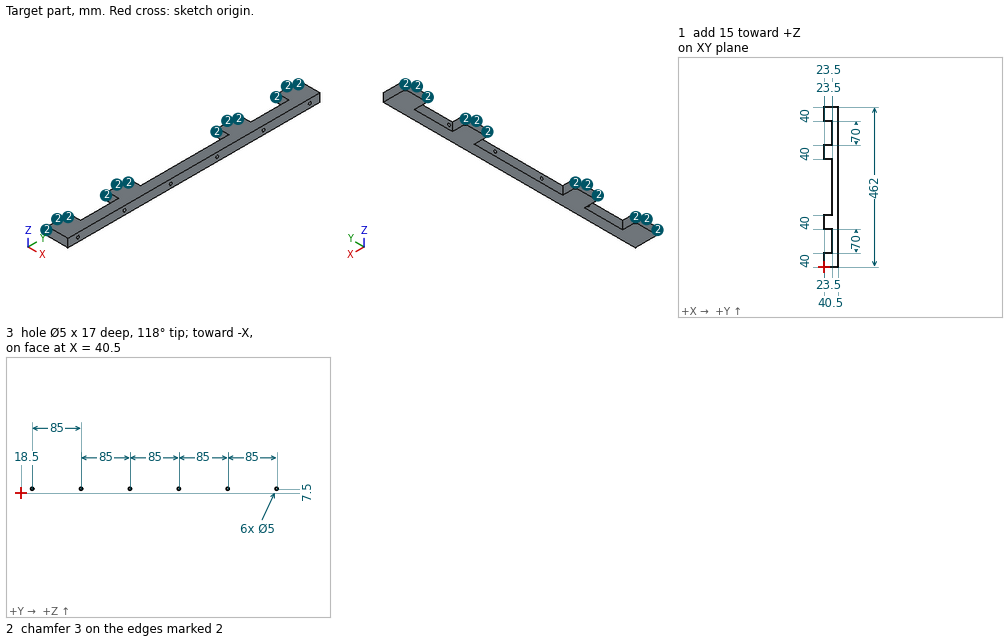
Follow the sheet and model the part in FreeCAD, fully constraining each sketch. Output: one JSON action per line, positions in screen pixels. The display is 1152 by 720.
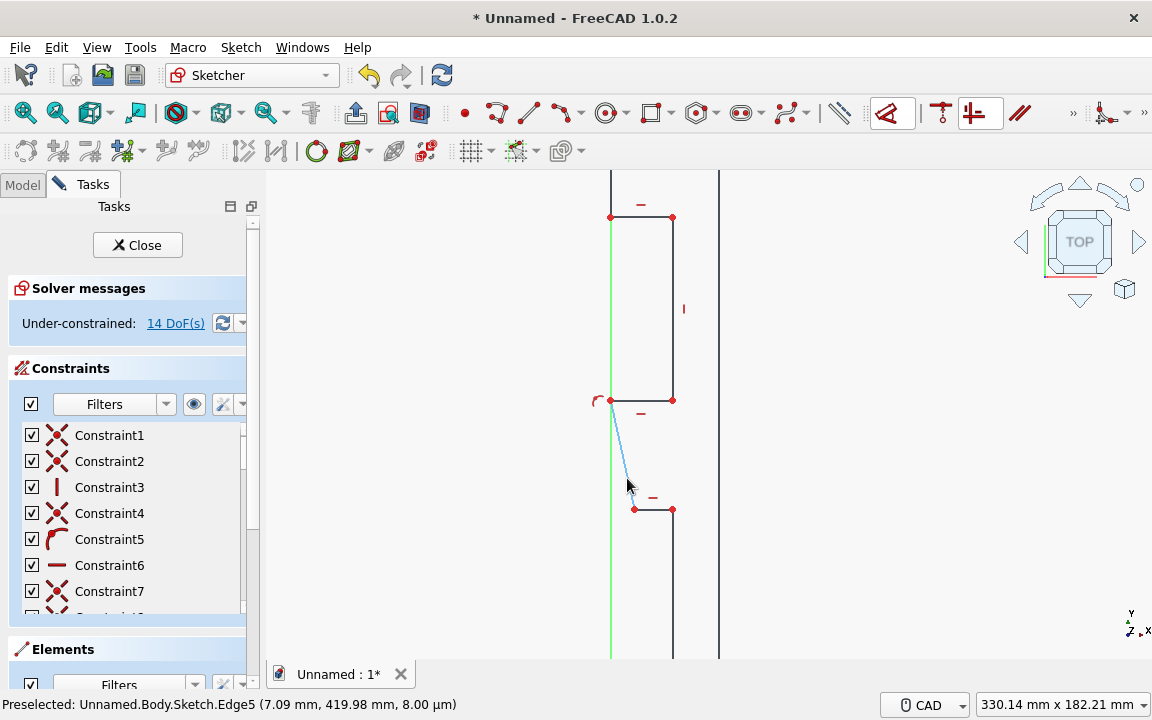
{"action": "left_click", "coordinate": [627, 477]}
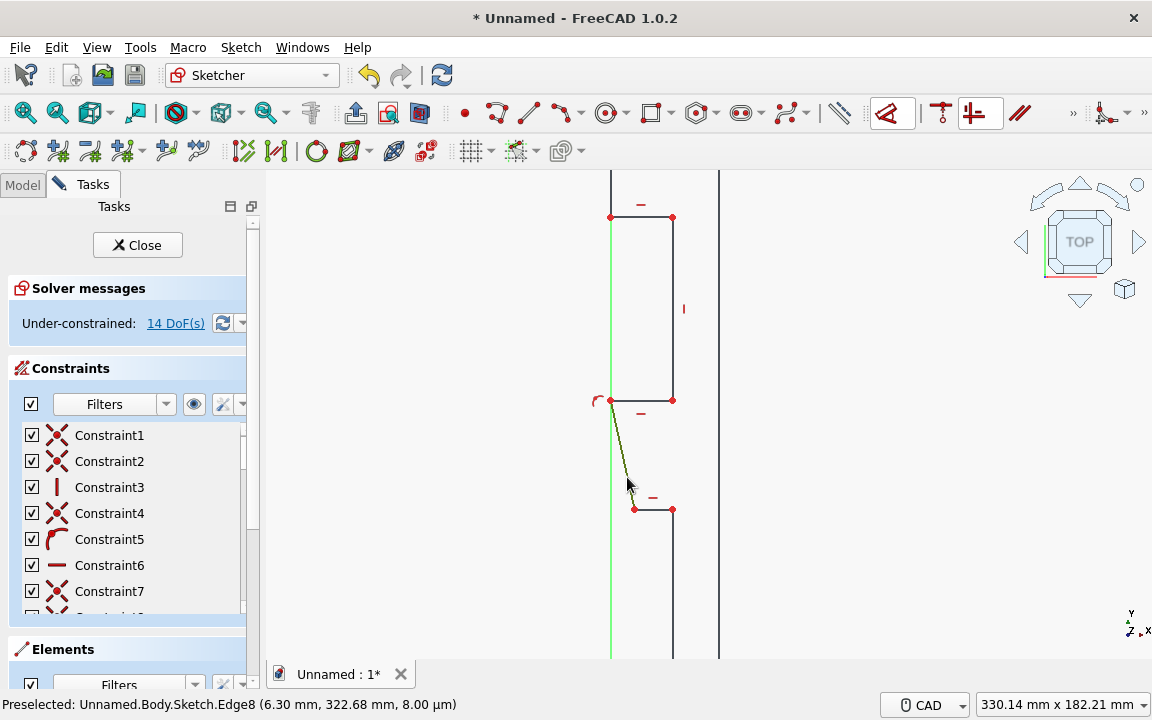
{"action": "key", "text": "v"}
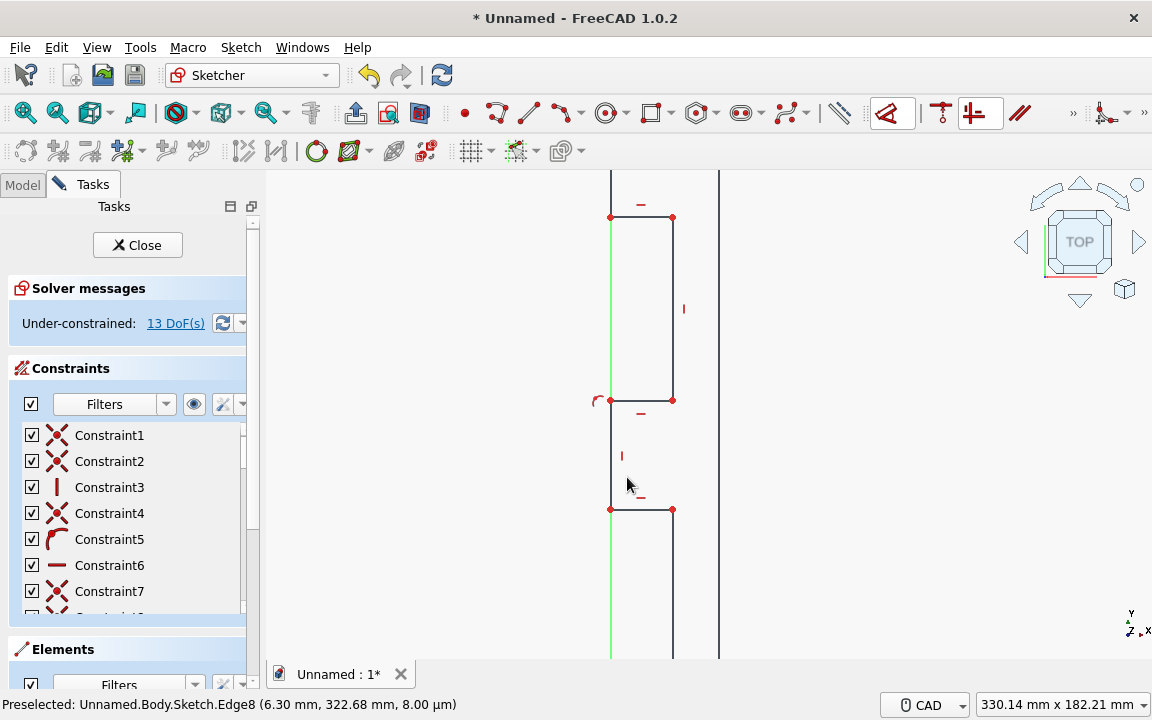
{"action": "scroll", "coordinate": [632, 313], "scroll_direction": "down", "scroll_amount": 7}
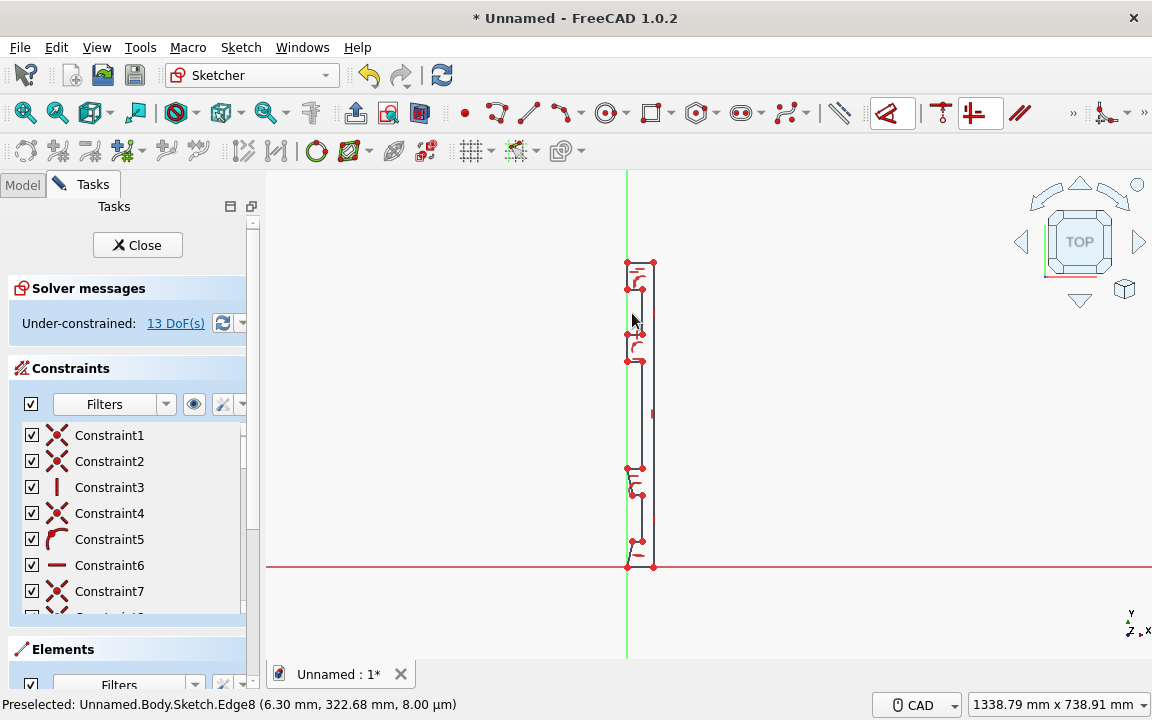
{"action": "scroll", "coordinate": [631, 487], "scroll_direction": "up", "scroll_amount": 7}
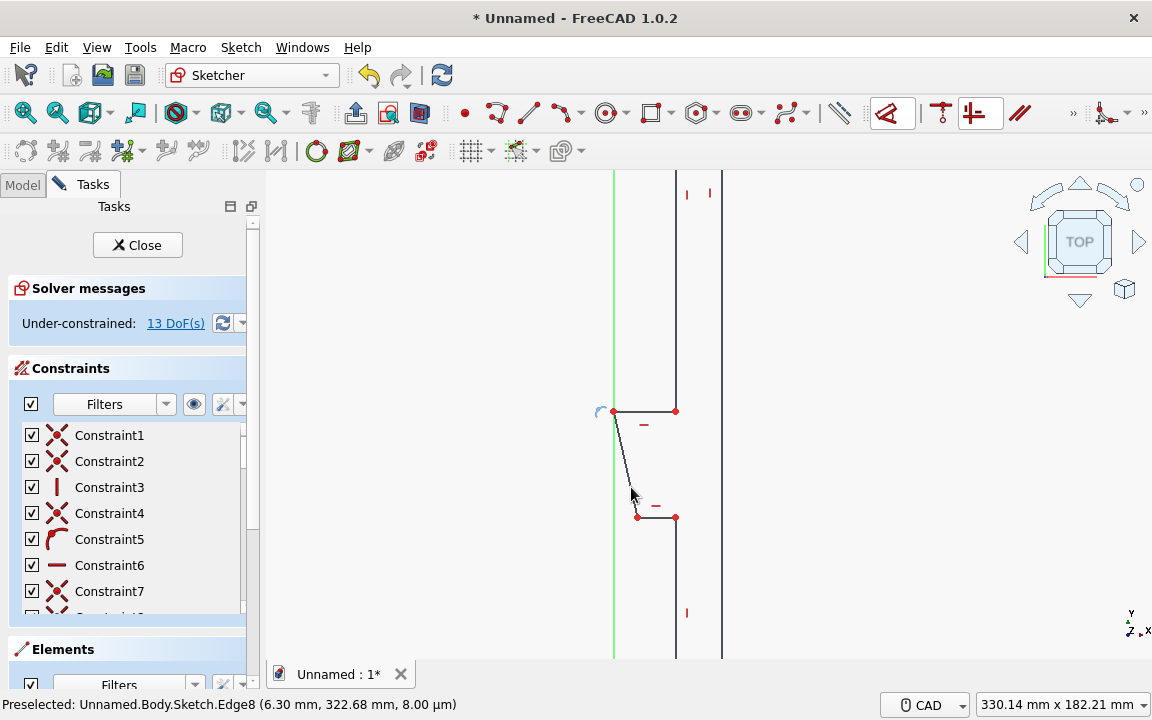
{"action": "left_click", "coordinate": [631, 486]}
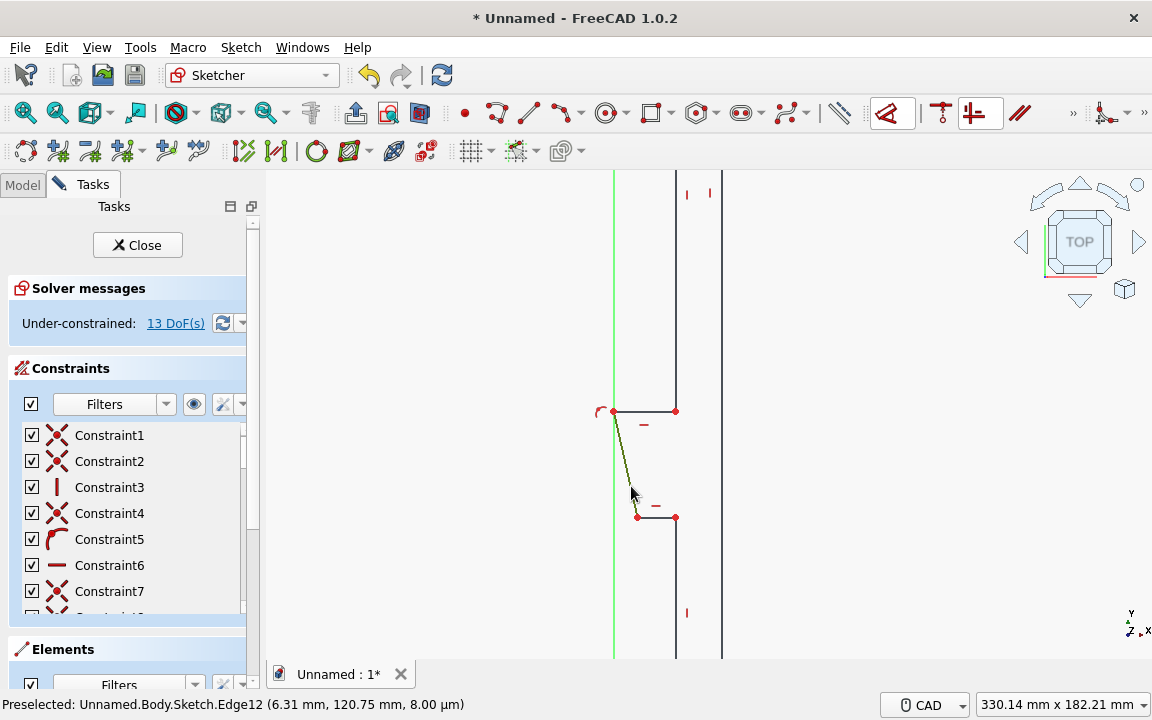
{"action": "left_click", "coordinate": [998, 114]}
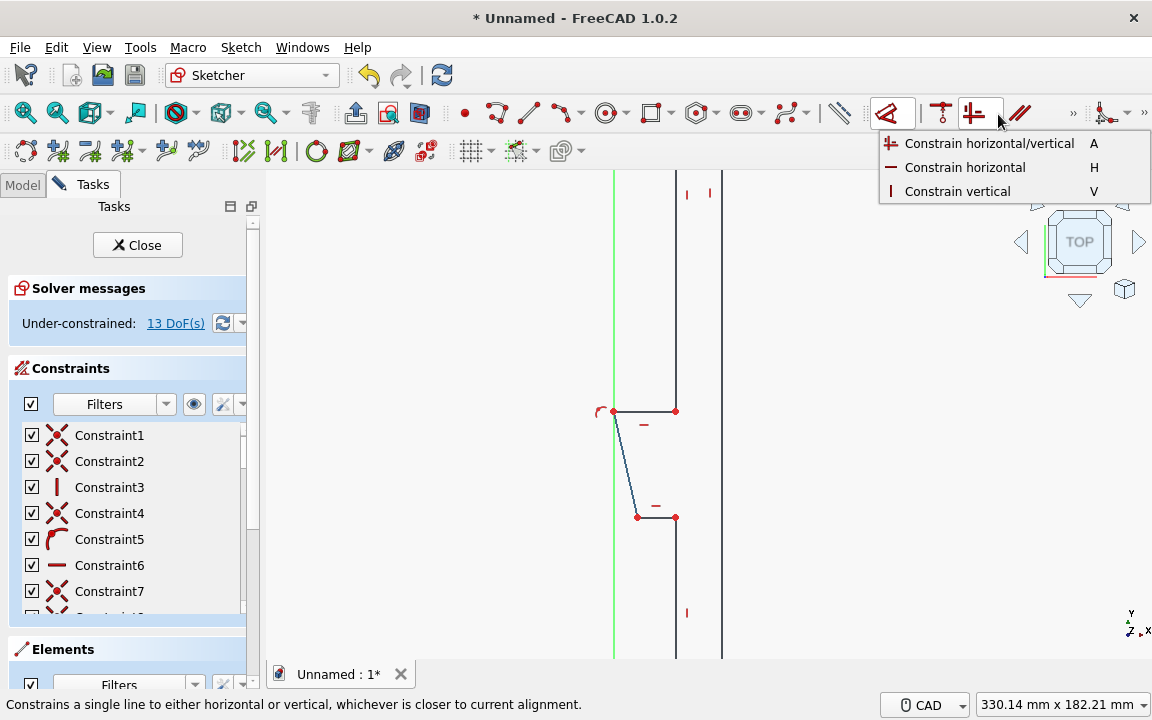
{"action": "left_click", "coordinate": [1015, 191]}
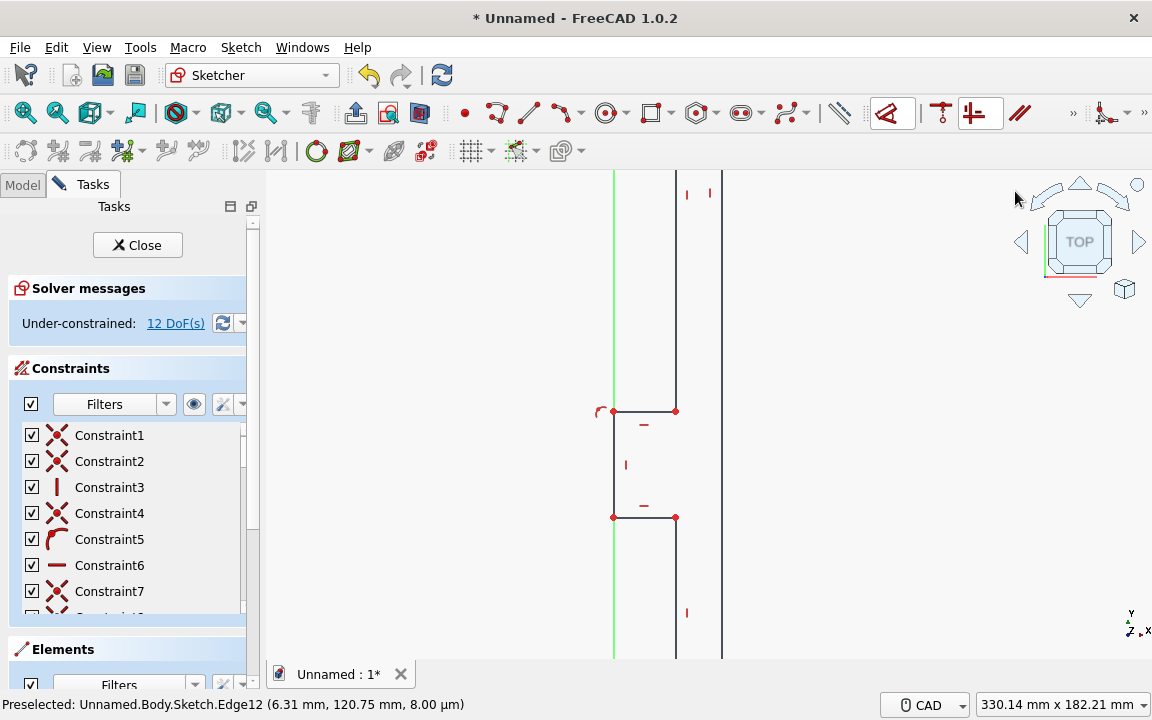
{"action": "scroll", "coordinate": [631, 488], "scroll_direction": "down", "scroll_amount": 7}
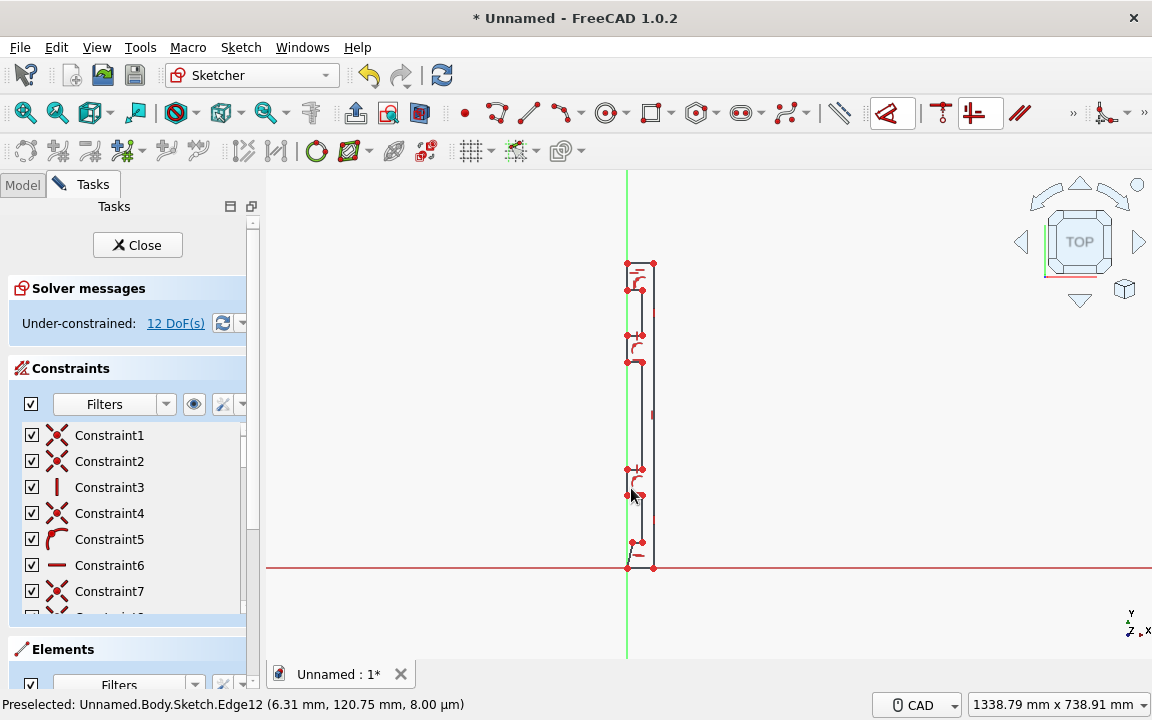
{"action": "scroll", "coordinate": [631, 550], "scroll_direction": "up", "scroll_amount": 7}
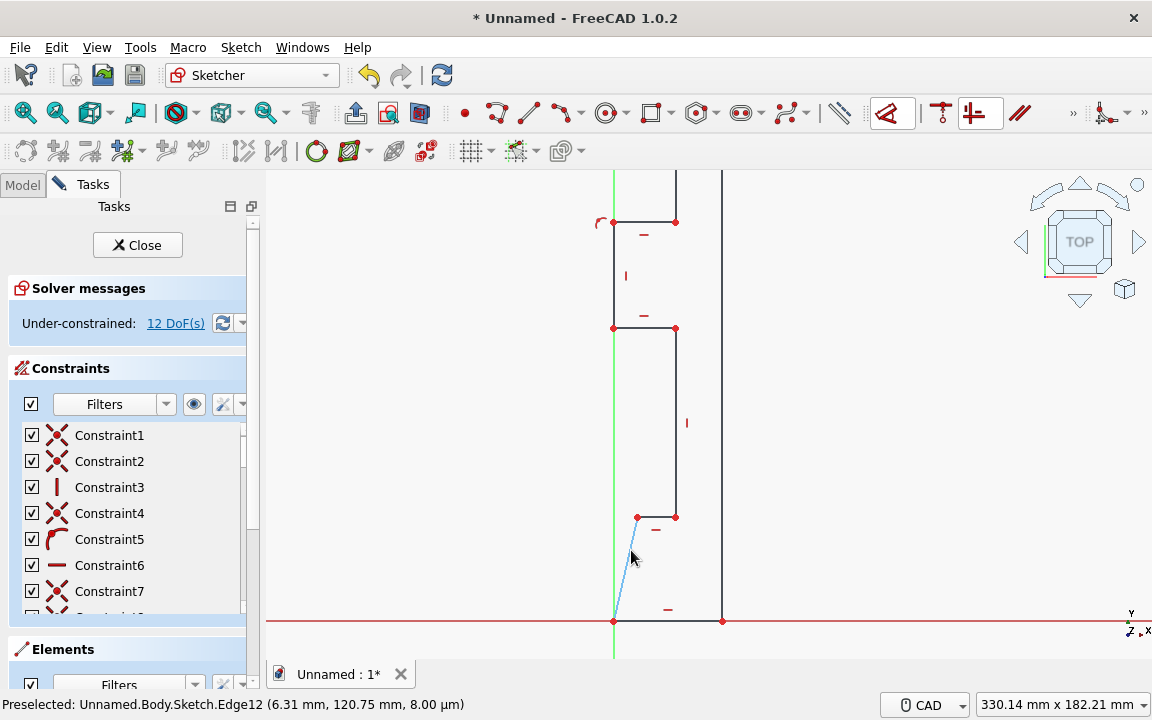
{"action": "left_click", "coordinate": [631, 549]}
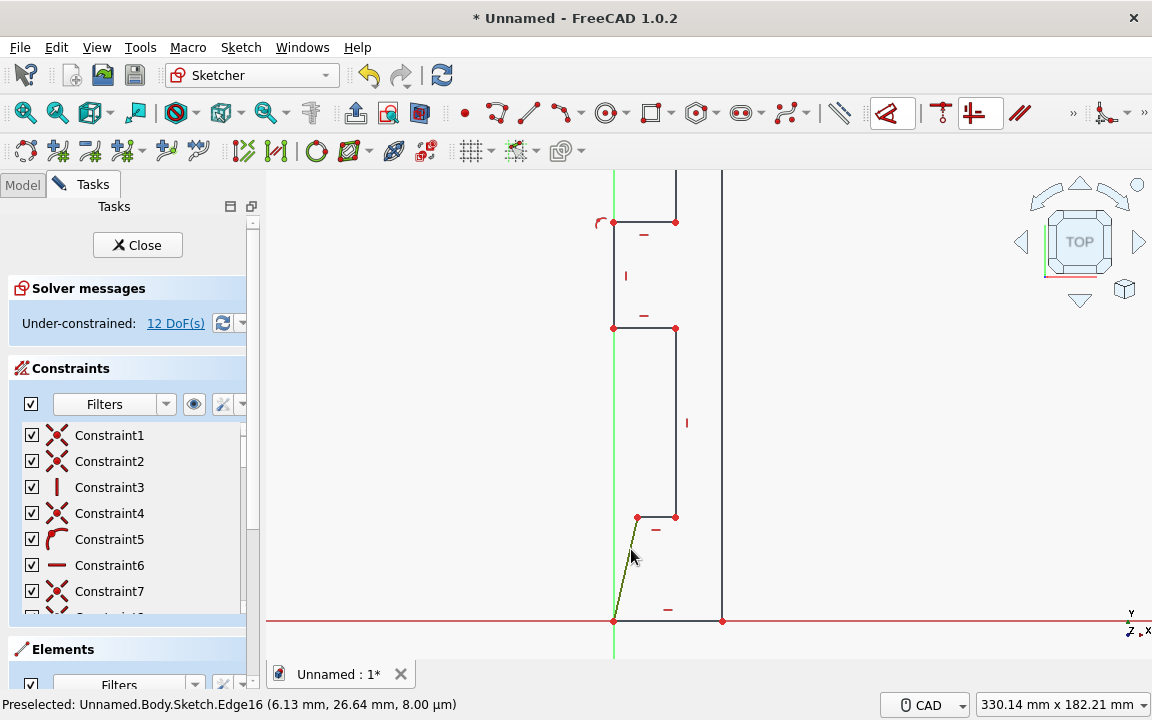
{"action": "key", "text": "v"}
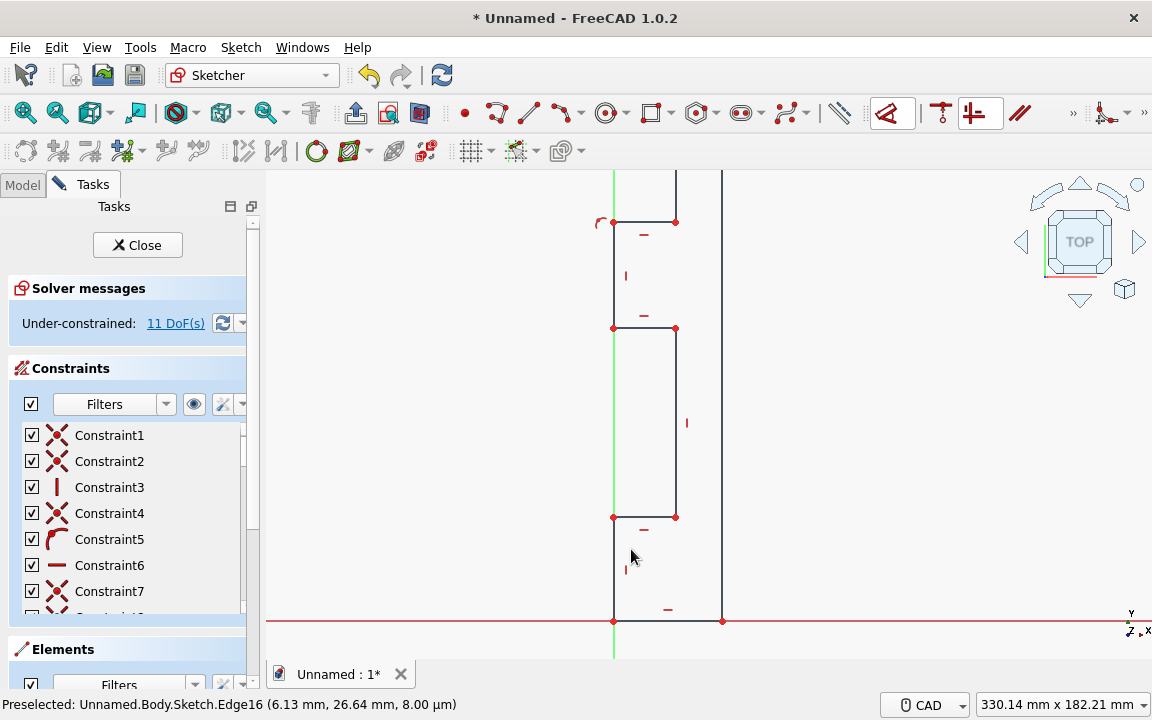
{"action": "left_click", "coordinate": [886, 114]}